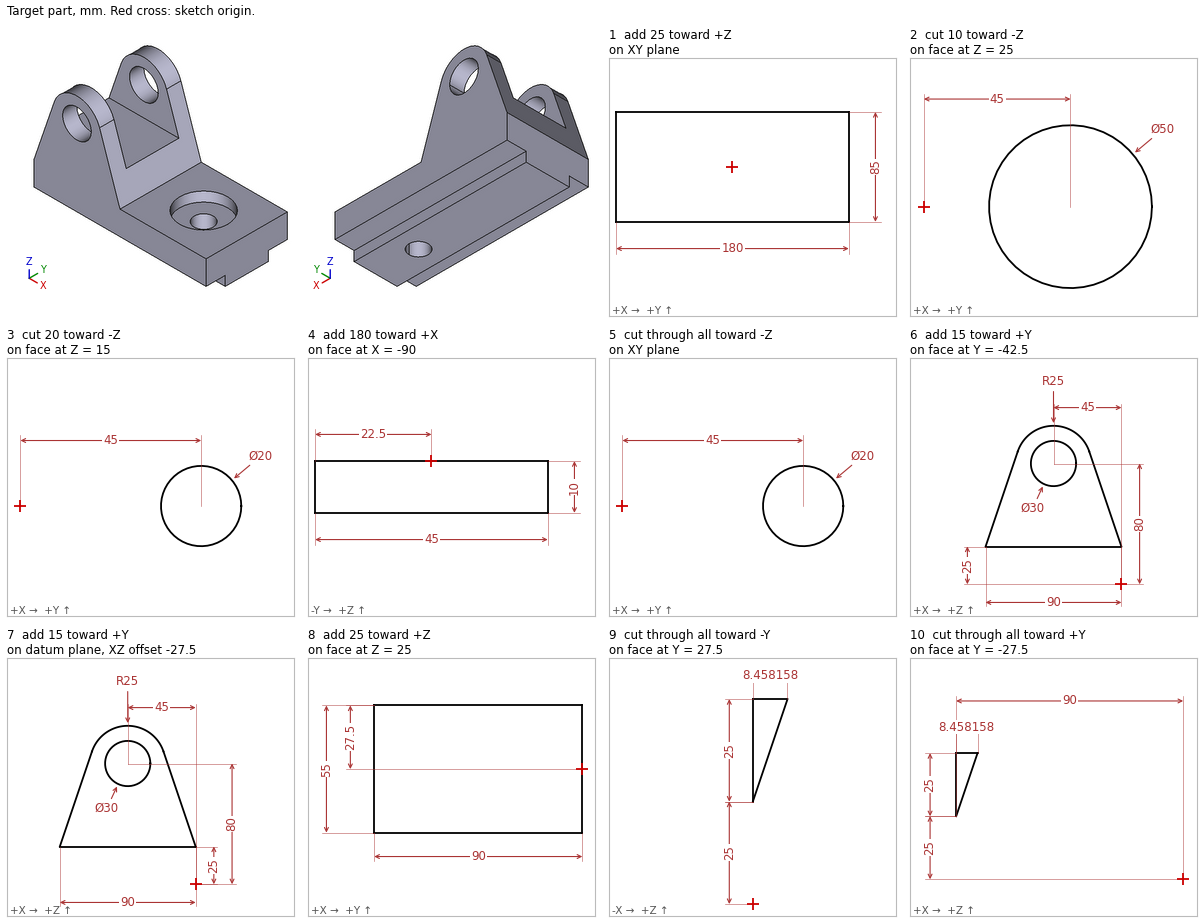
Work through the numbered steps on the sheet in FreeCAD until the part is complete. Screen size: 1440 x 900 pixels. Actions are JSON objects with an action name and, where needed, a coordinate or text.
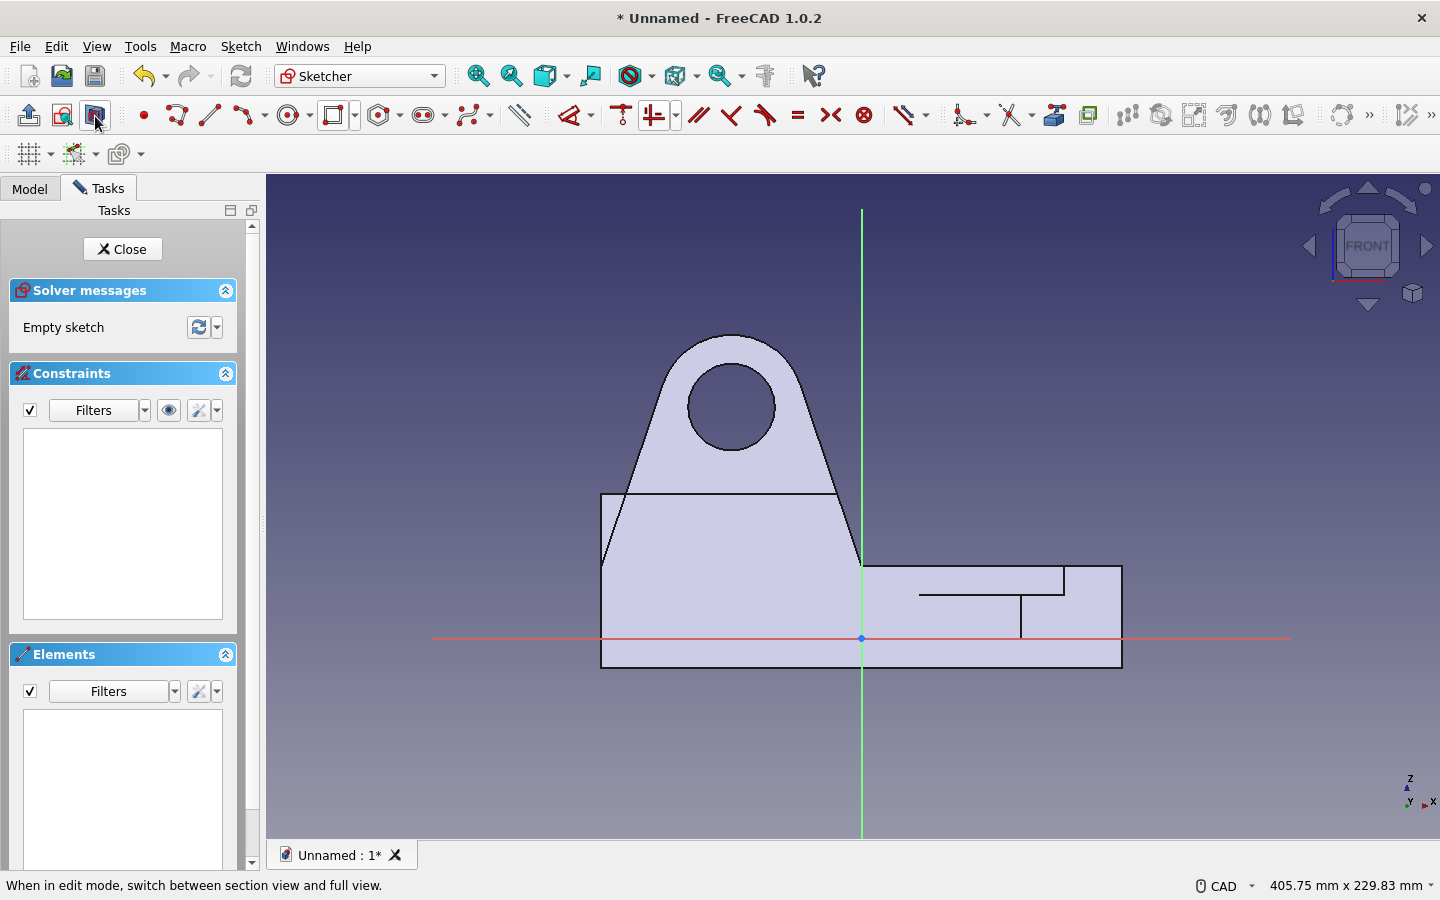
{"action": "scroll", "coordinate": [580, 535], "scroll_direction": "up", "scroll_amount": 9}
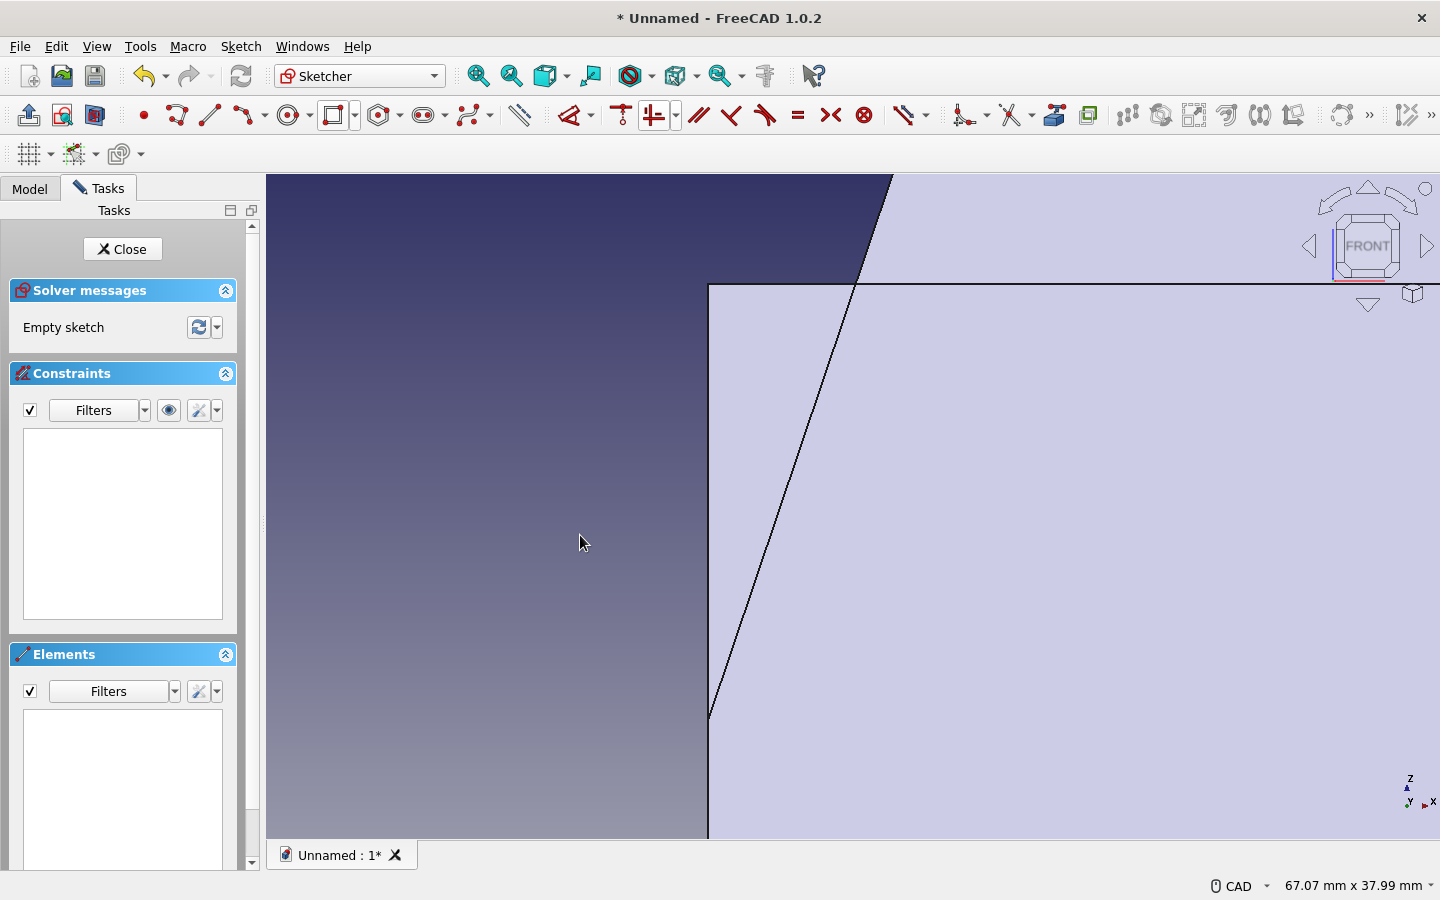
{"action": "left_click", "coordinate": [177, 116]}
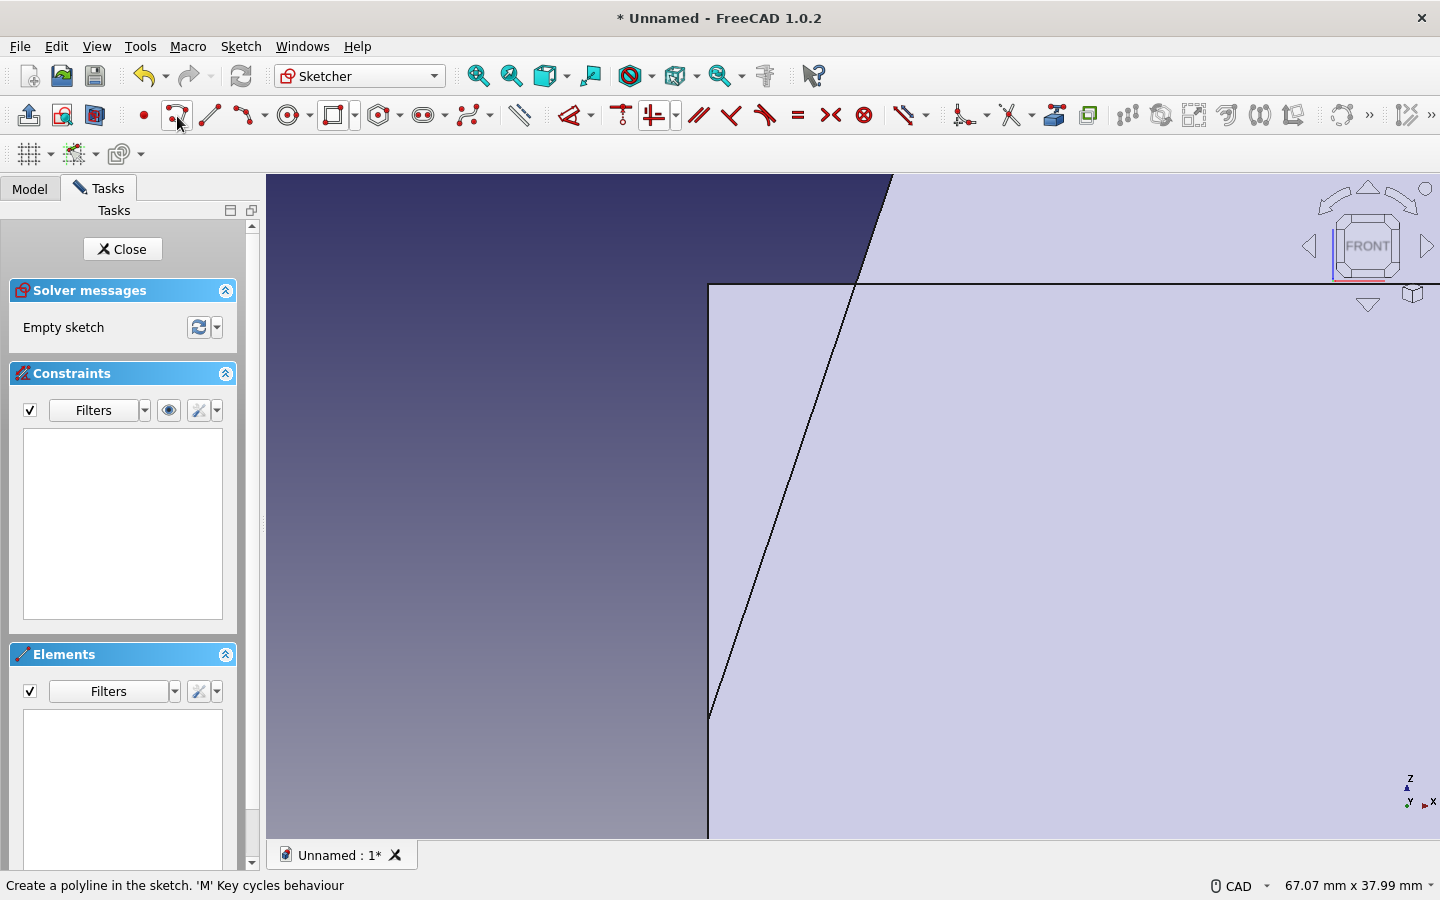
{"action": "left_click", "coordinate": [708, 721]}
{"action": "left_click", "coordinate": [856, 284]}
{"action": "left_click", "coordinate": [708, 284]}
{"action": "left_click", "coordinate": [708, 722]}
{"action": "key", "text": "Escape"}
{"action": "key", "text": "Escape"}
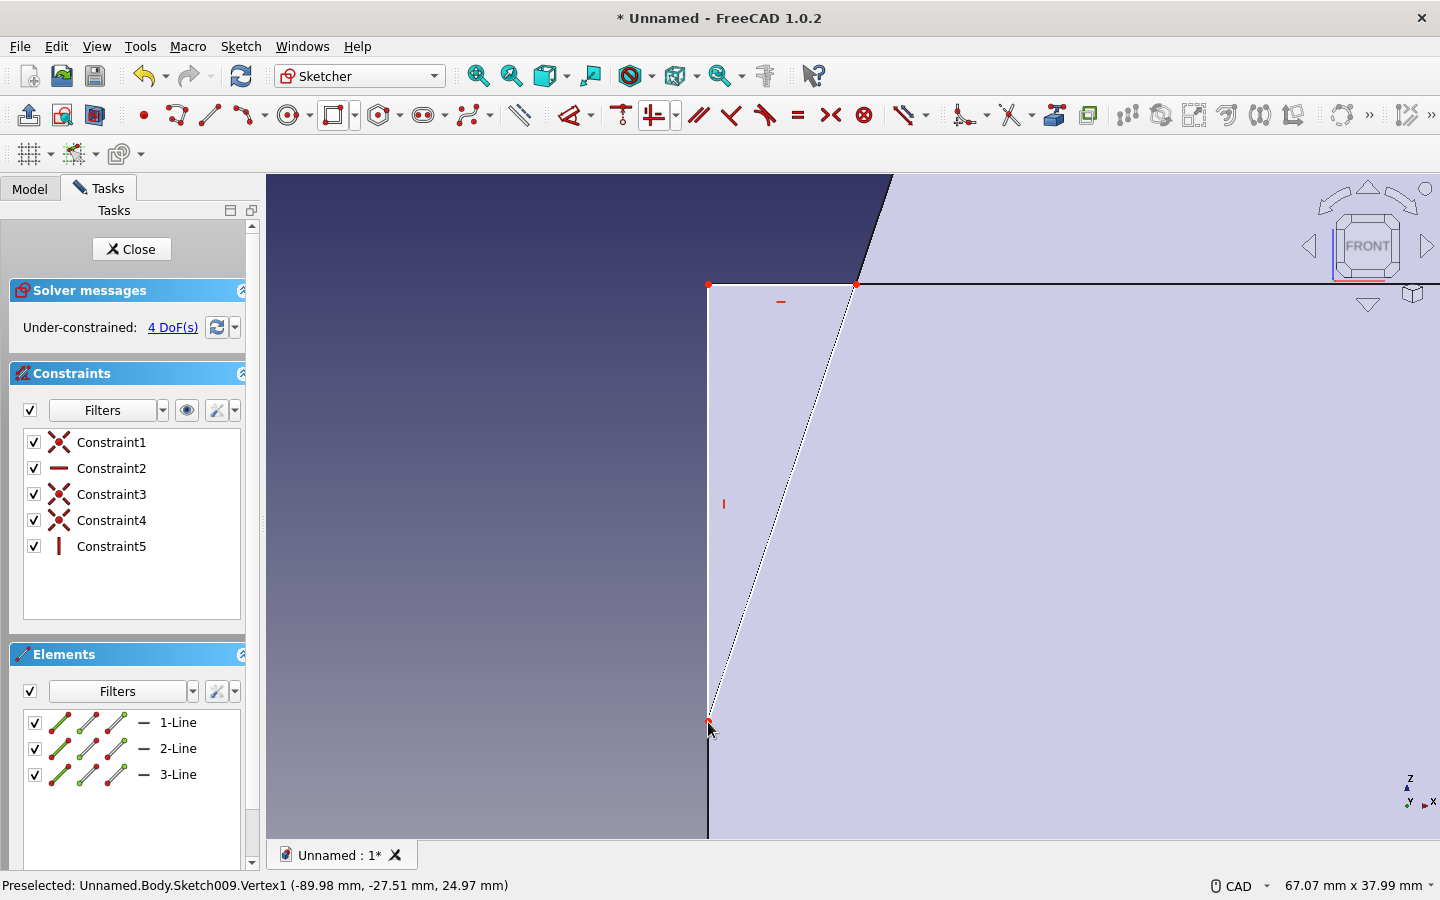
{"action": "left_click", "coordinate": [568, 116]}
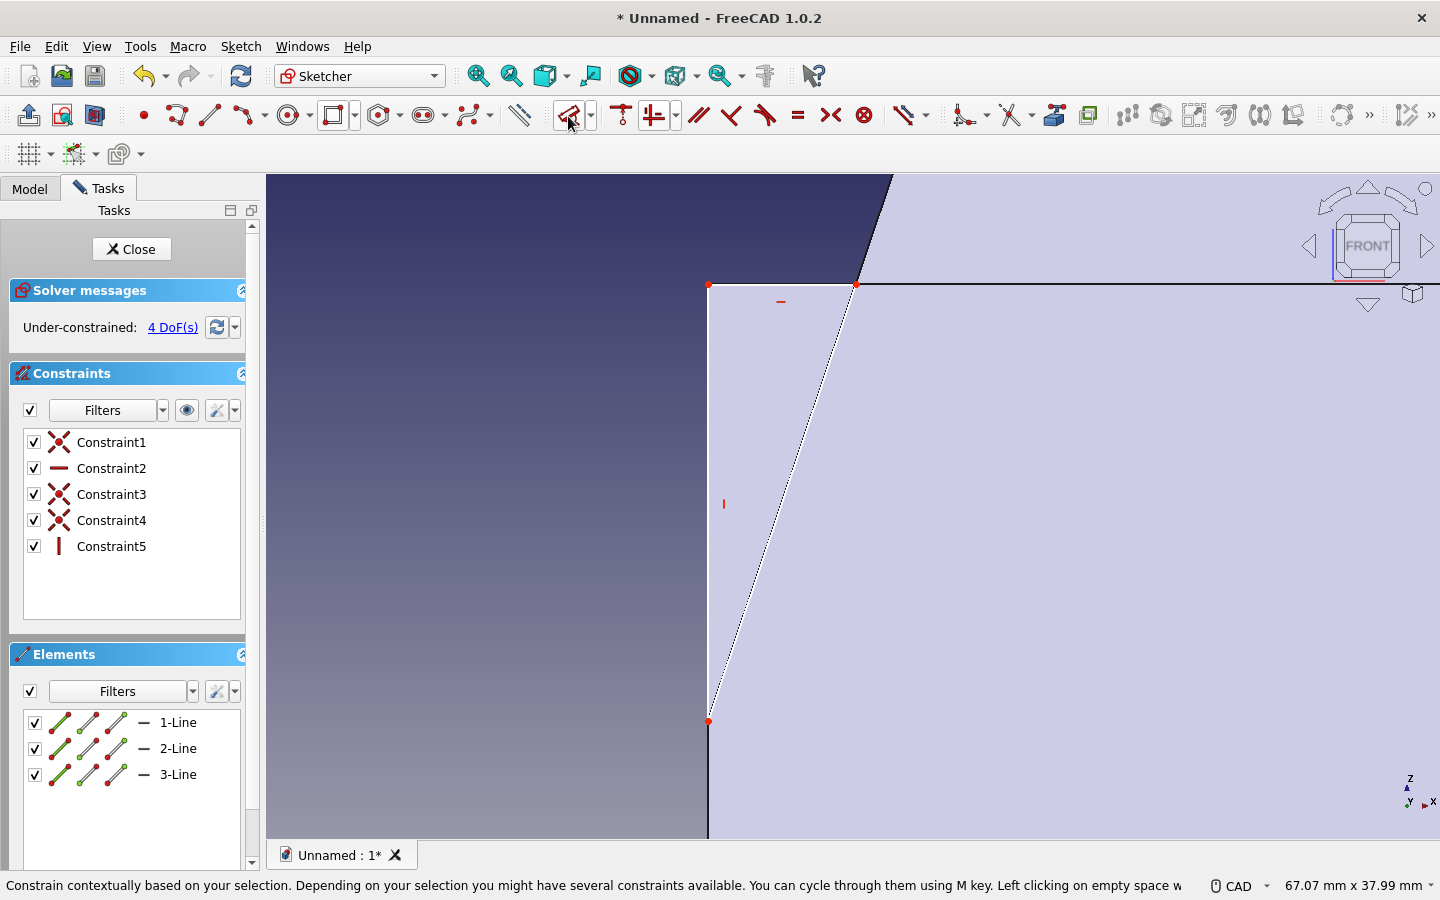
{"action": "left_click", "coordinate": [708, 416]}
{"action": "left_click", "coordinate": [674, 503]}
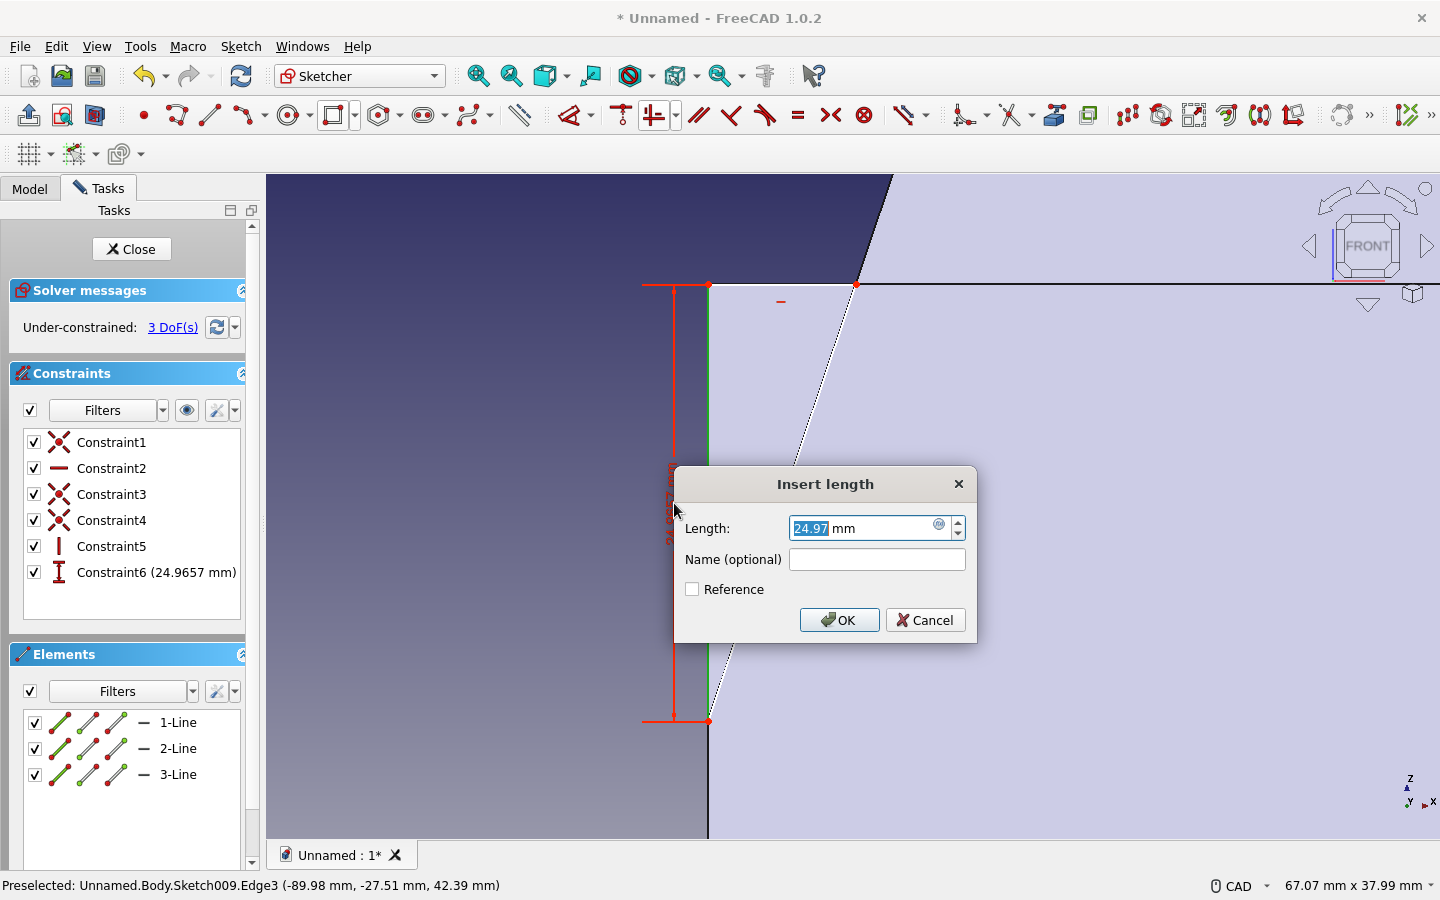
{"action": "type", "text": "25"}
{"action": "key", "text": "Return"}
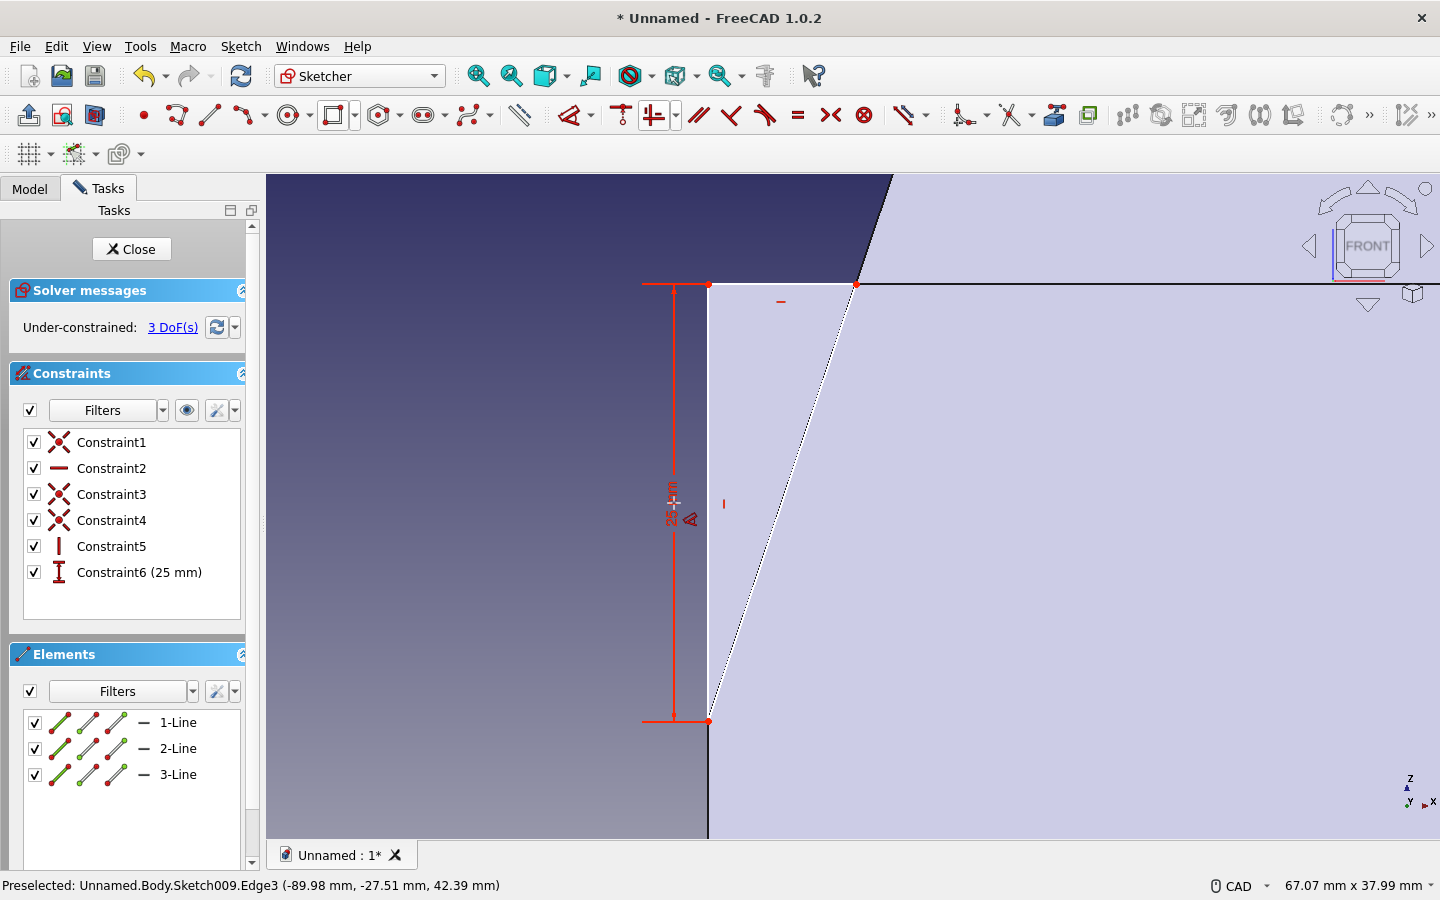
{"action": "left_click", "coordinate": [708, 722]}
{"action": "left_click", "coordinate": [991, 688]}